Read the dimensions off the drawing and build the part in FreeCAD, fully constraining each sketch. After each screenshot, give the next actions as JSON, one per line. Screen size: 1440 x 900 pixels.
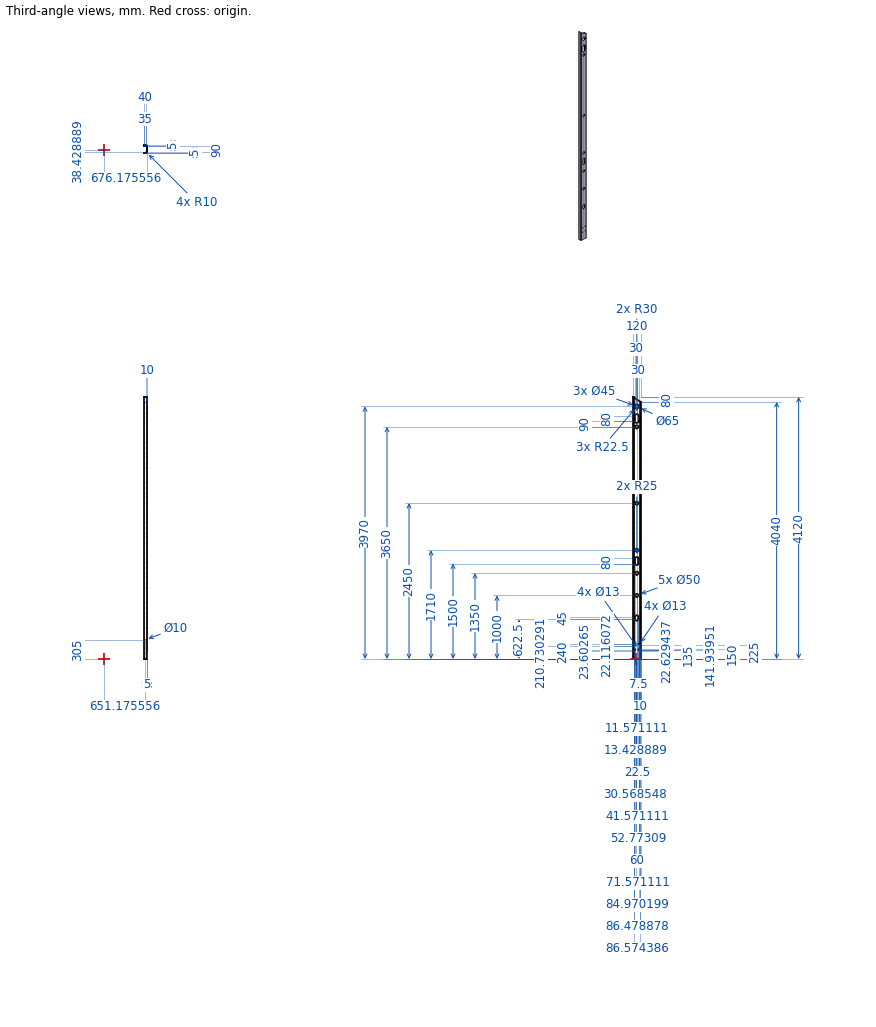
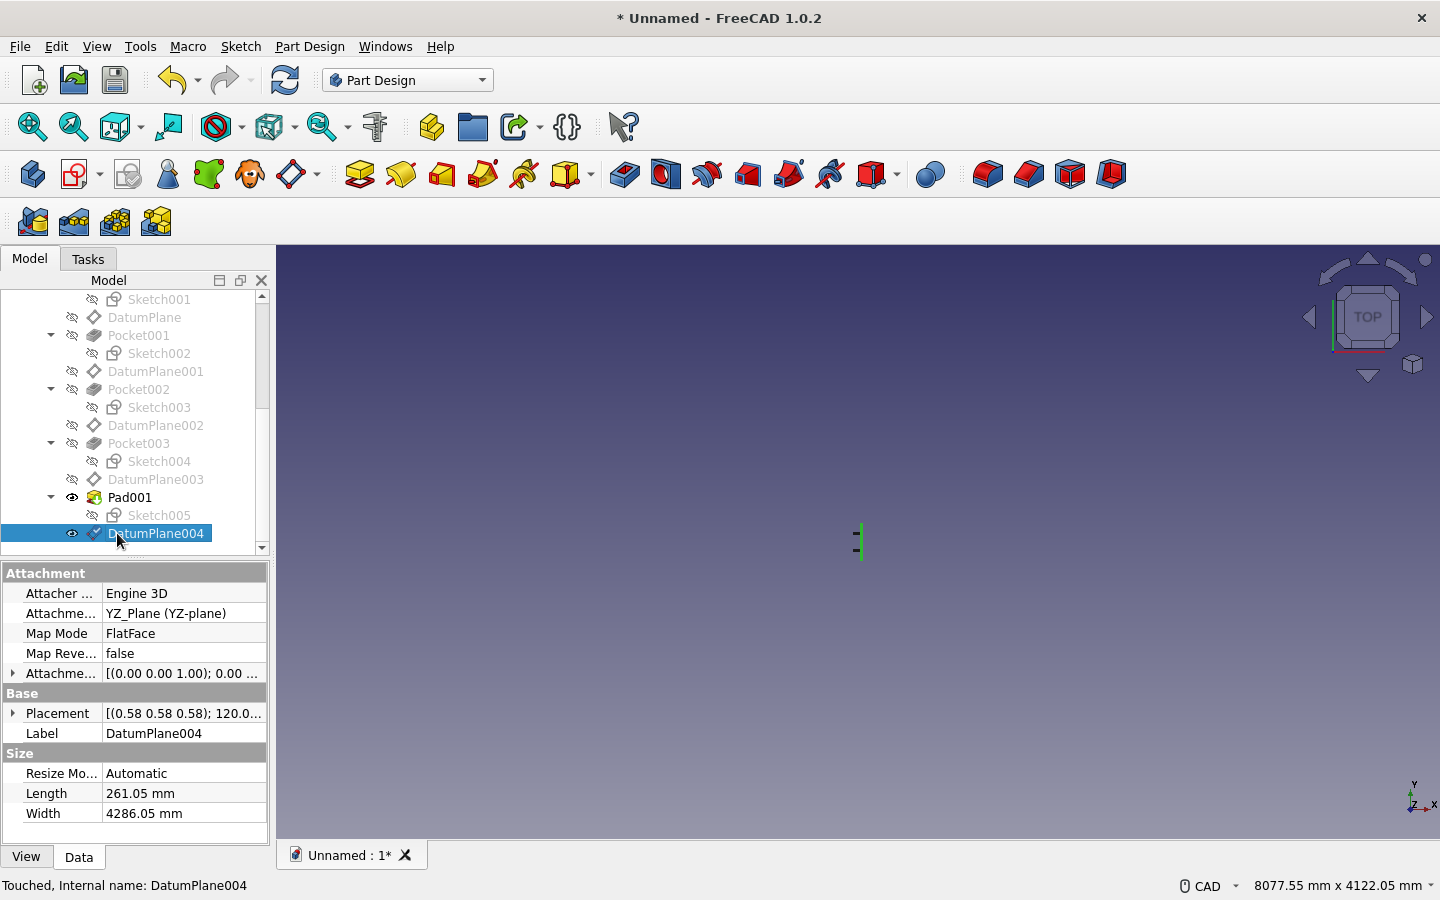
{"action": "left_click", "coordinate": [74, 174]}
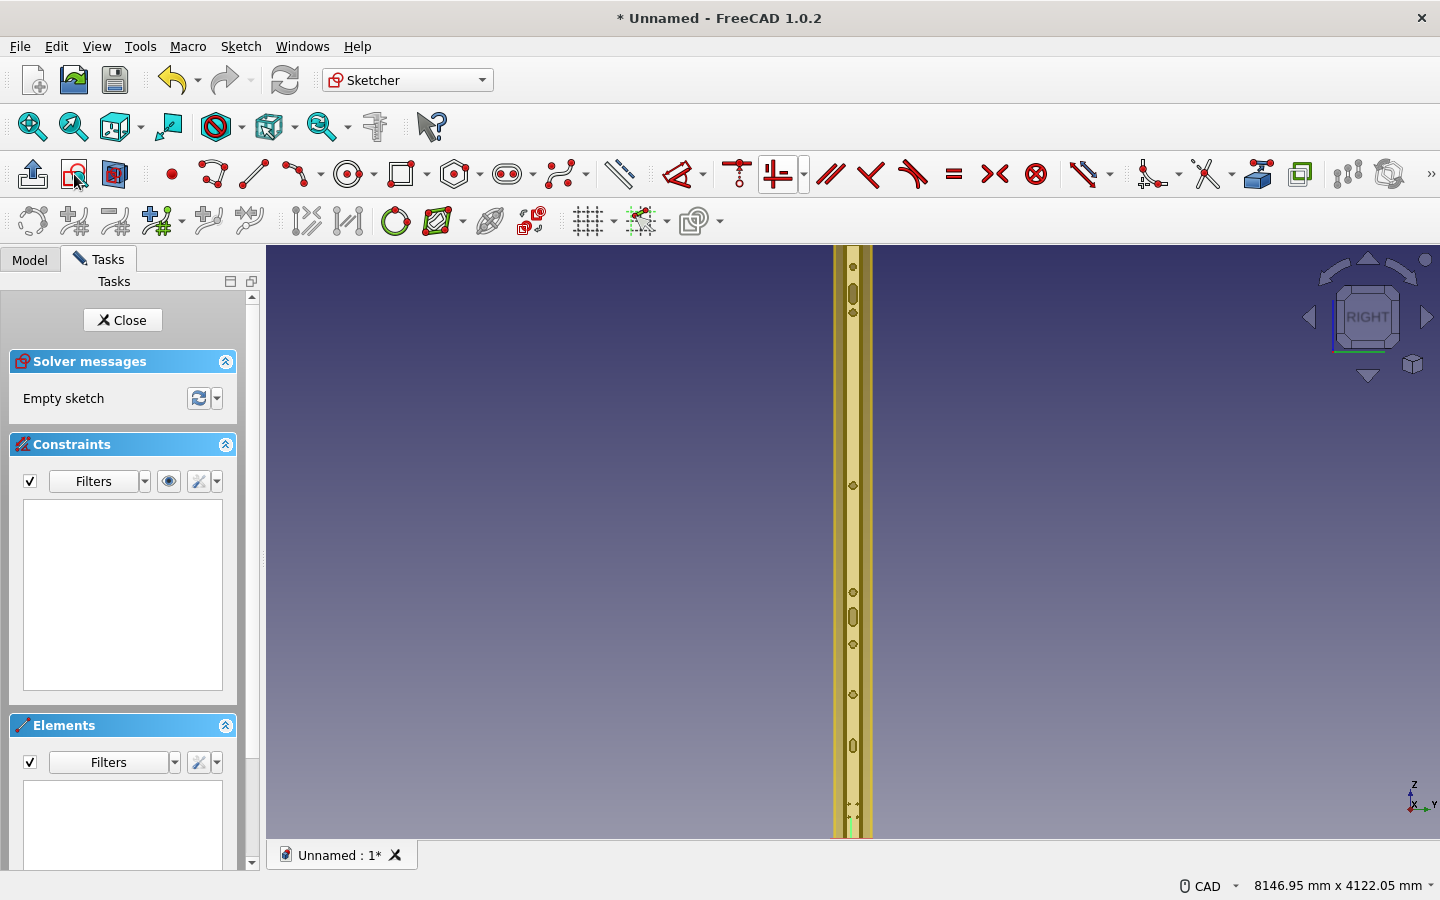
{"action": "scroll", "coordinate": [784, 542], "scroll_direction": "down", "scroll_amount": 5}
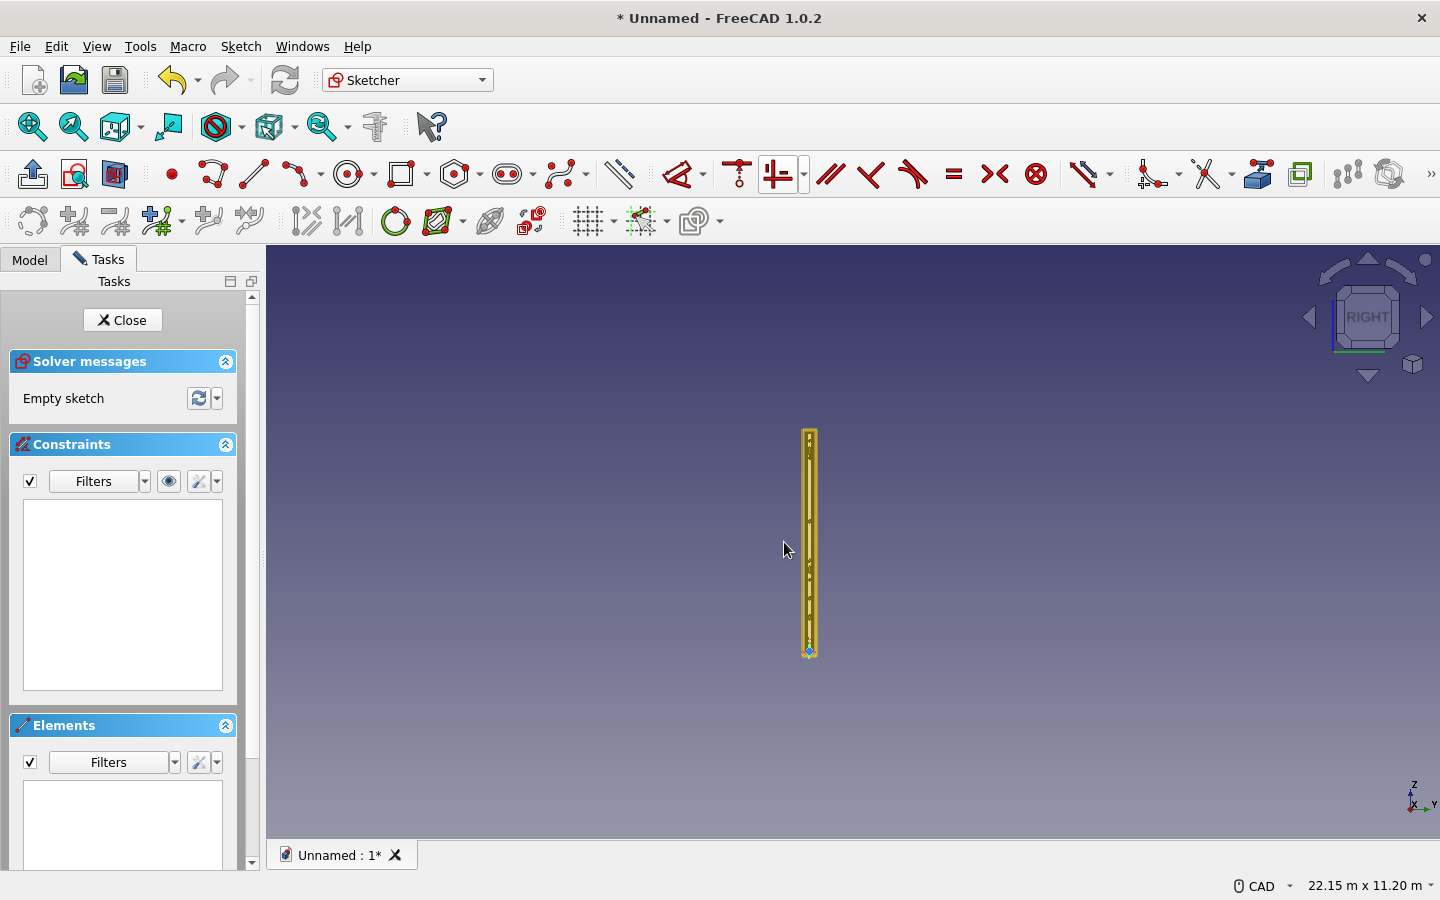
{"action": "scroll", "coordinate": [811, 436], "scroll_direction": "up", "scroll_amount": 15}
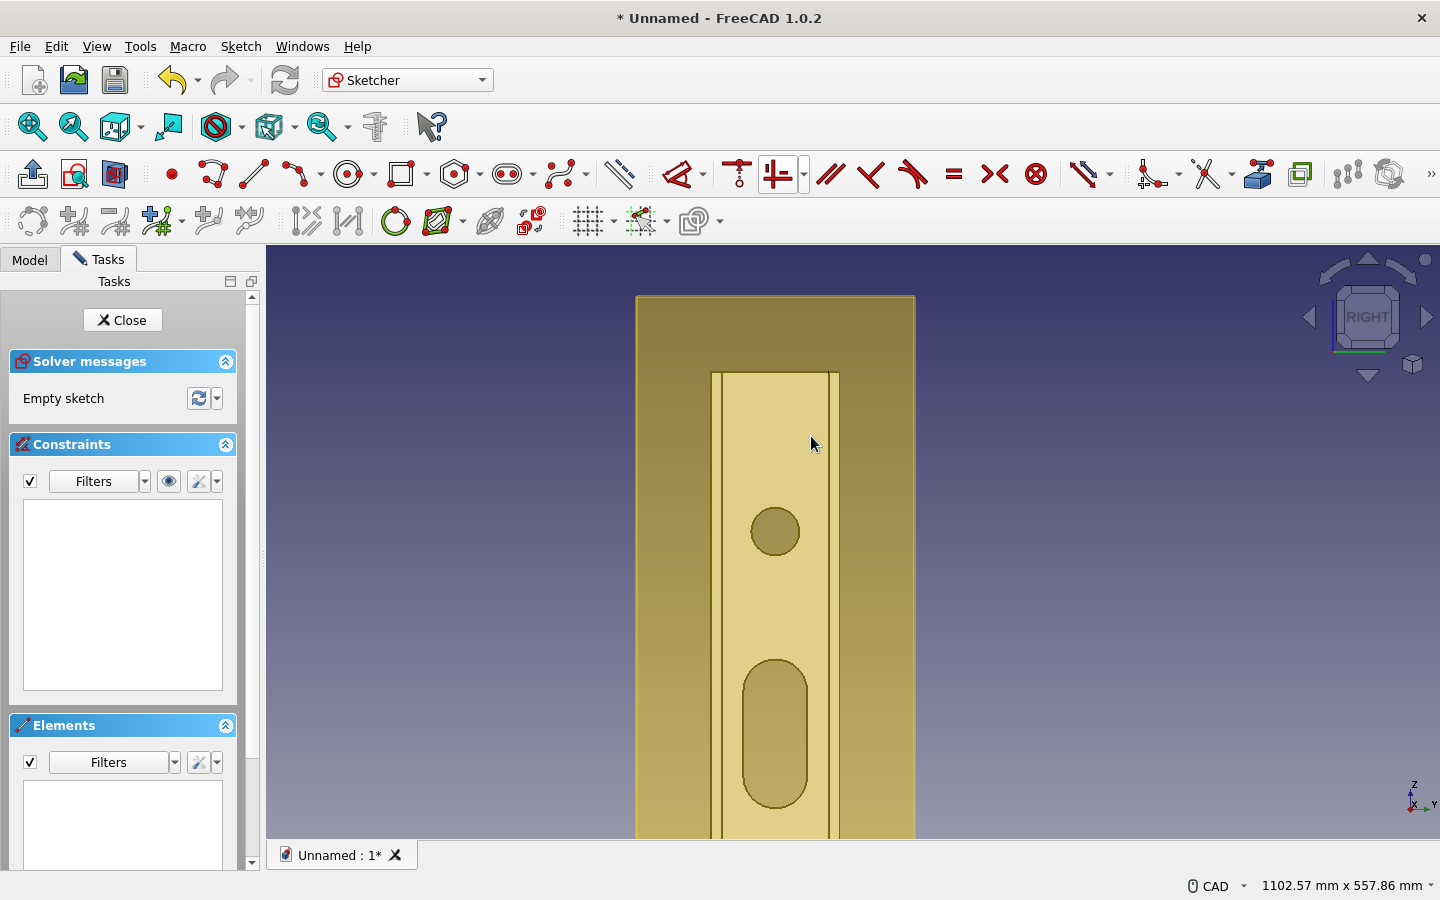
{"action": "scroll", "coordinate": [773, 529], "scroll_direction": "up", "scroll_amount": 9}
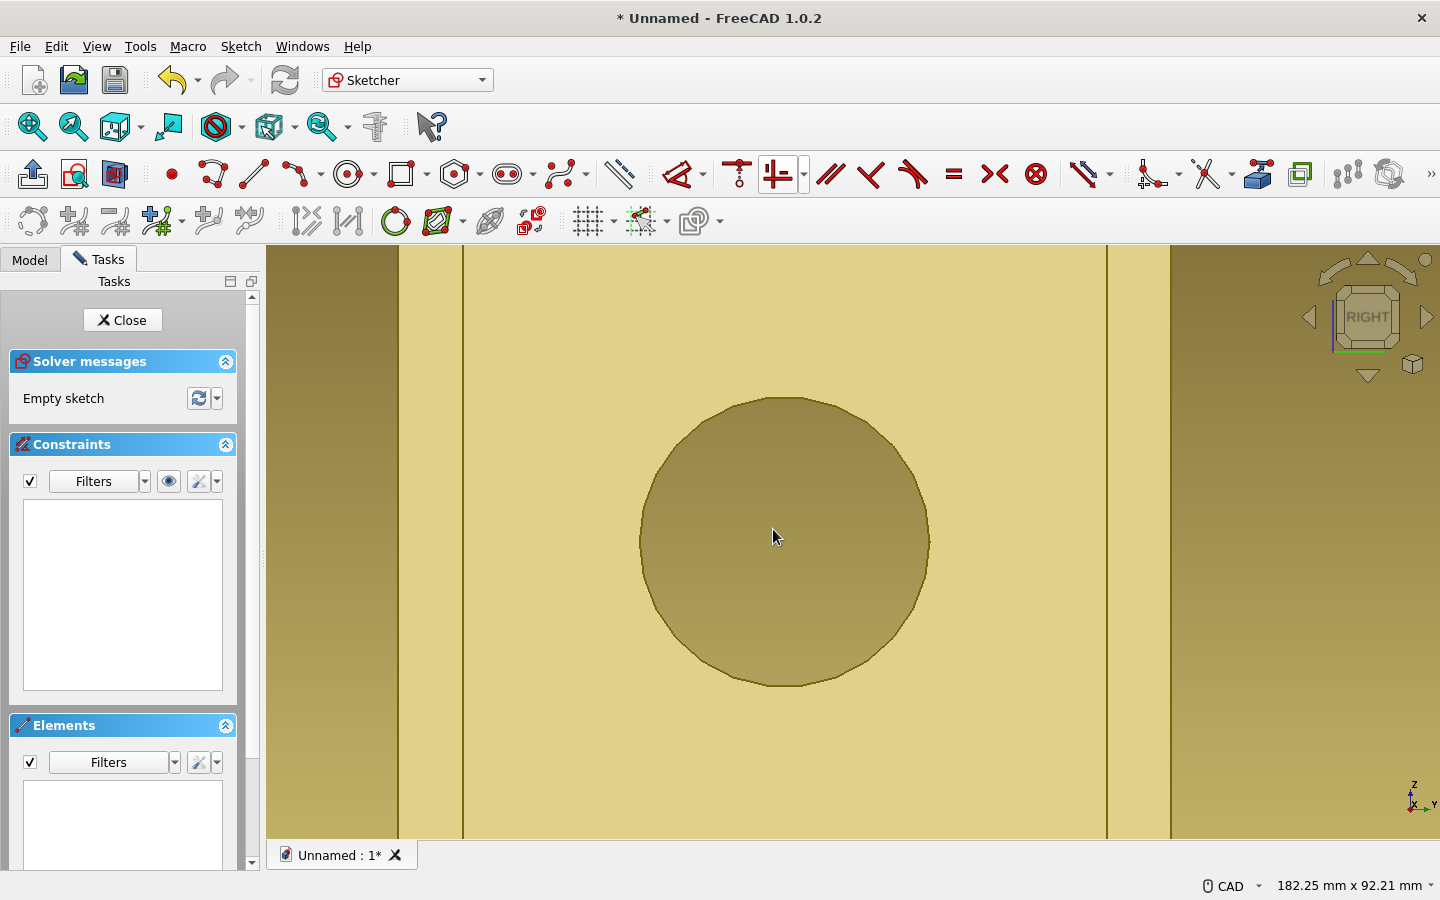
{"action": "key", "text": "g c"}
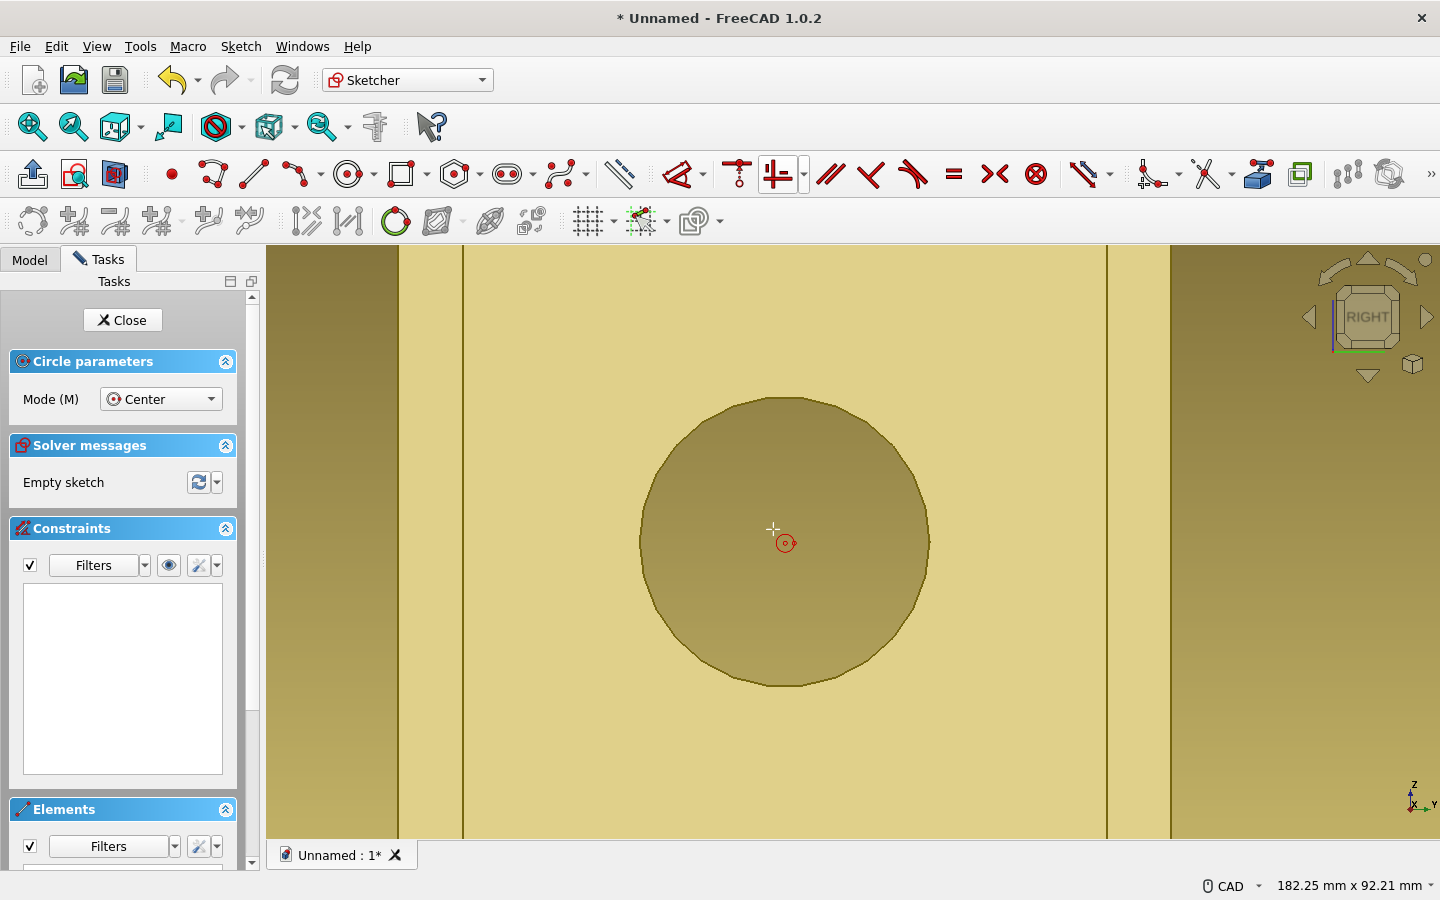
{"action": "left_click", "coordinate": [785, 542]}
{"action": "mouse_move", "coordinate": [933, 394]}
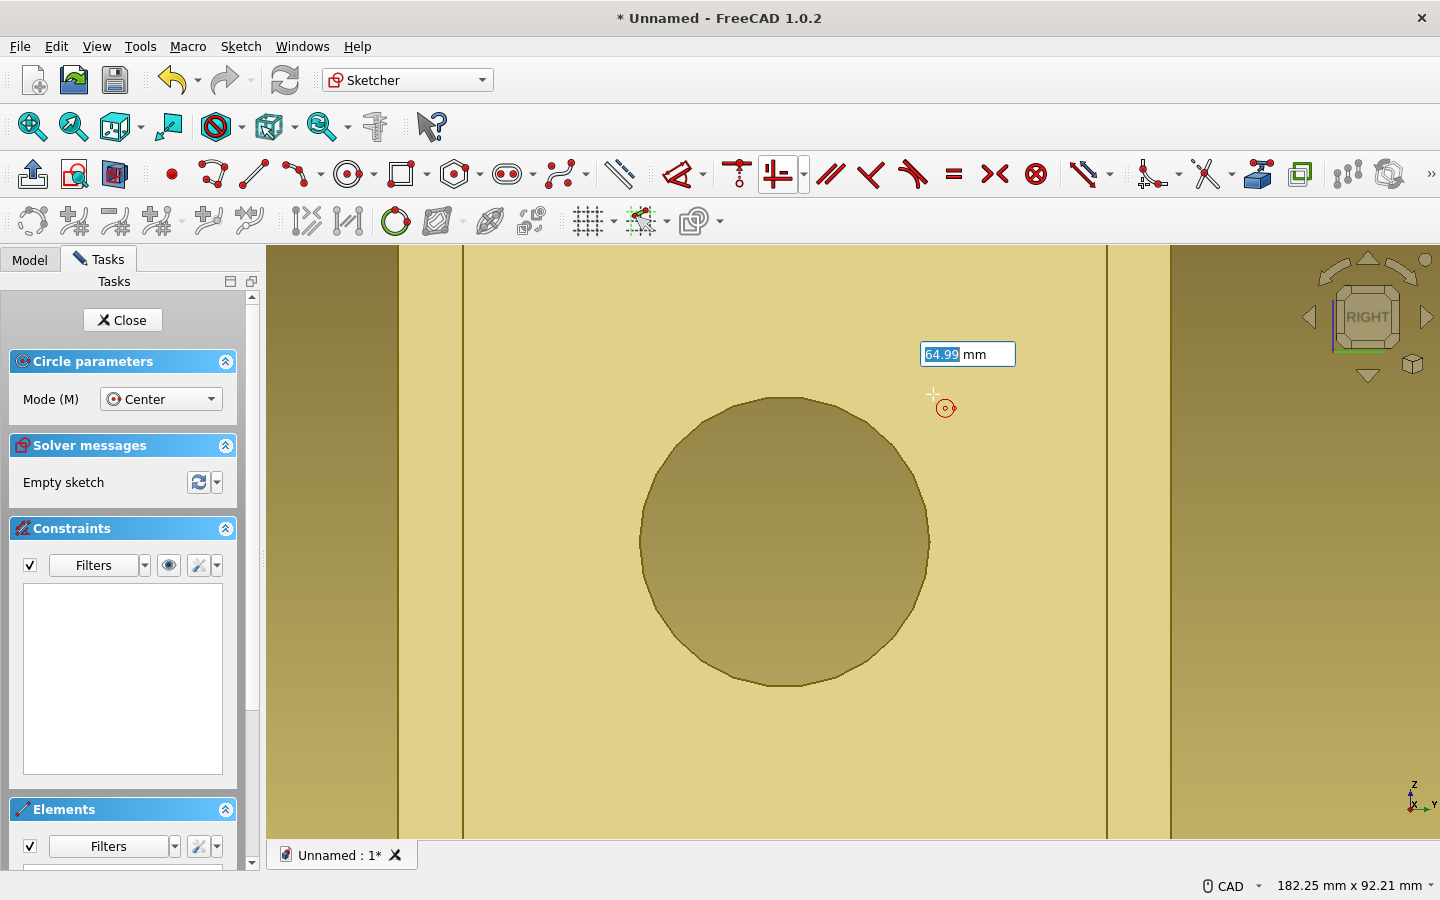
{"action": "type", "text": "65"}
{"action": "key", "text": "Return"}
{"action": "key", "text": "Escape"}